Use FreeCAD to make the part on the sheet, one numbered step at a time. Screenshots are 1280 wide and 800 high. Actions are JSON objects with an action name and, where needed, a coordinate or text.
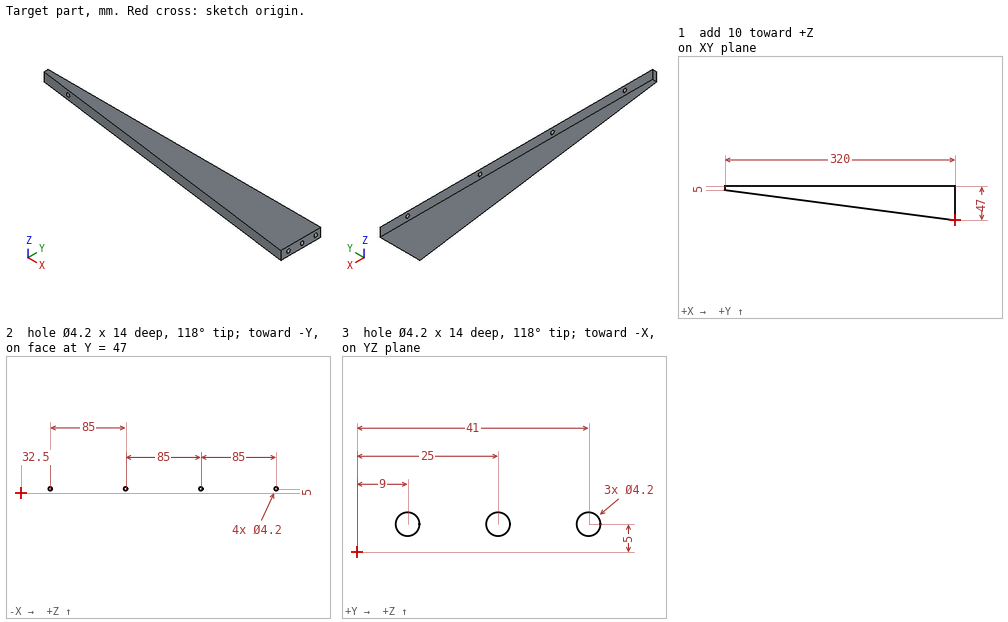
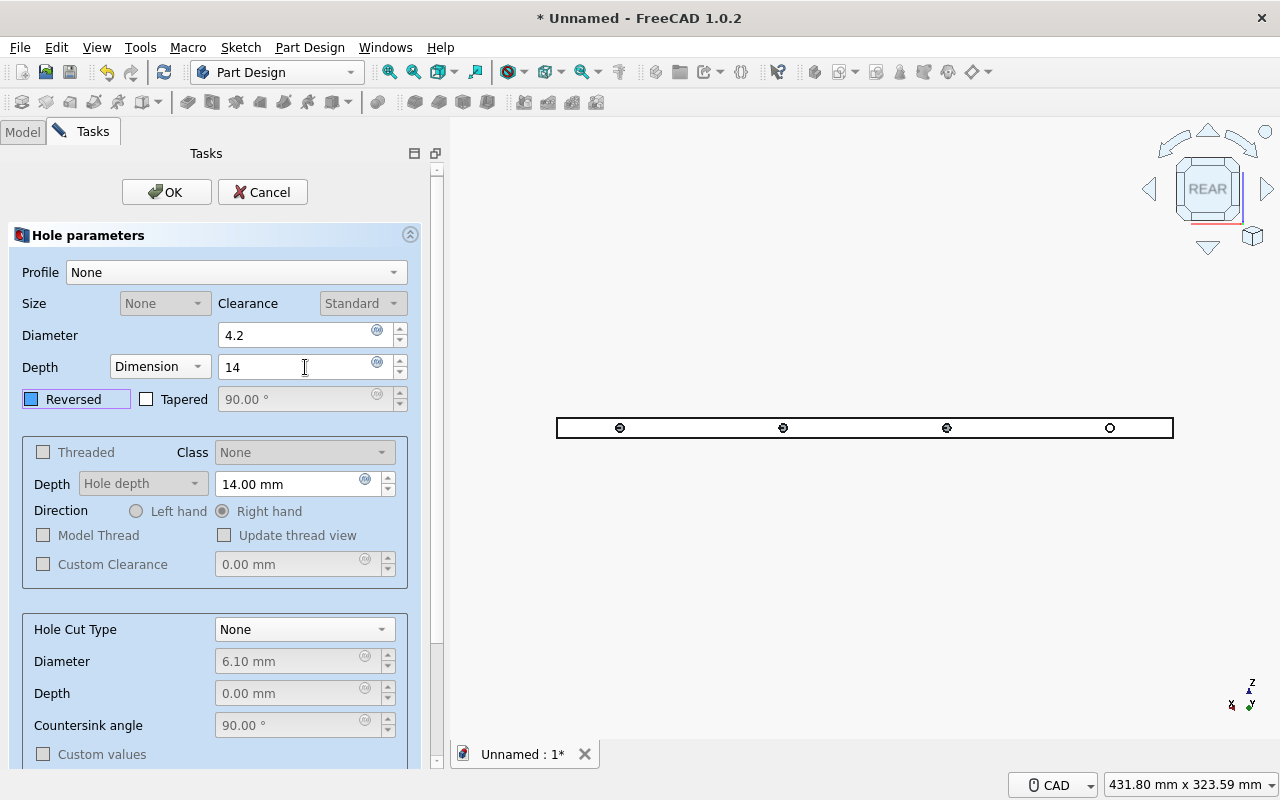
{"action": "left_click", "coordinate": [167, 192]}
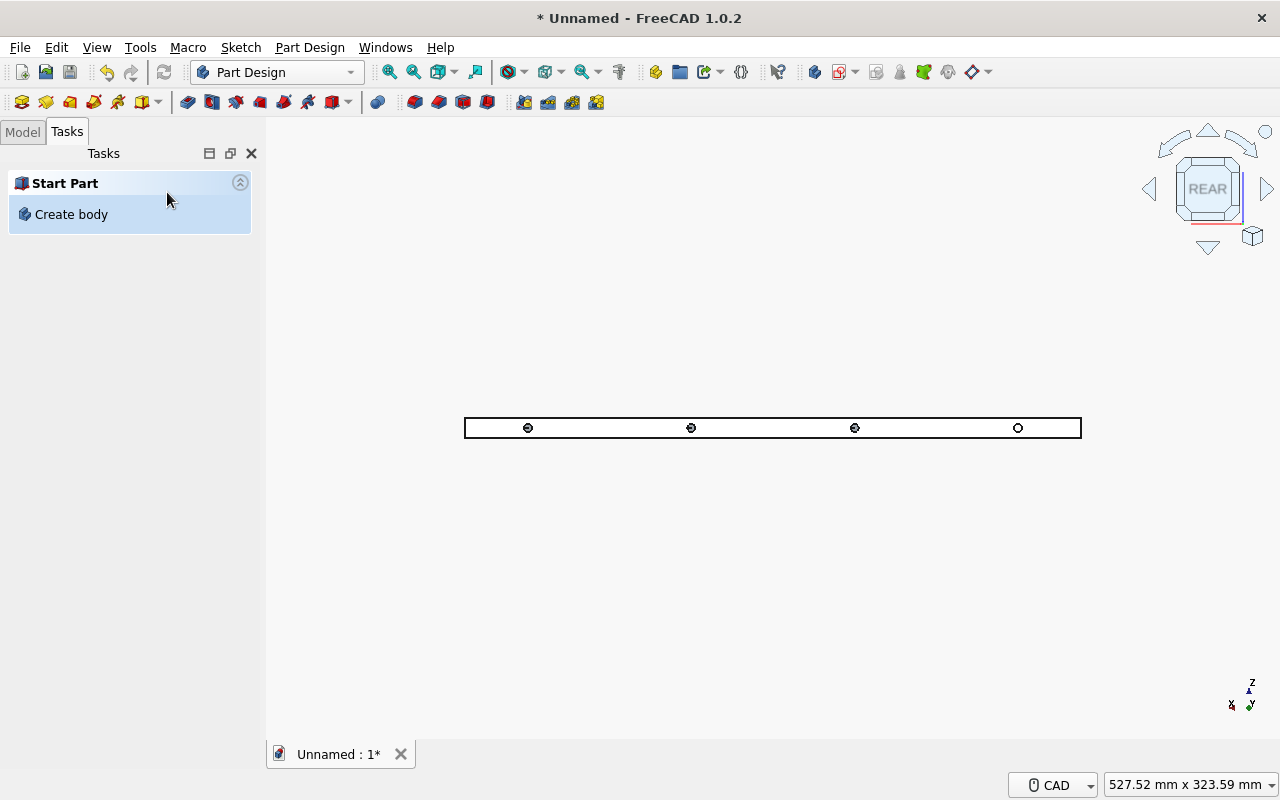
{"action": "key", "text": "0"}